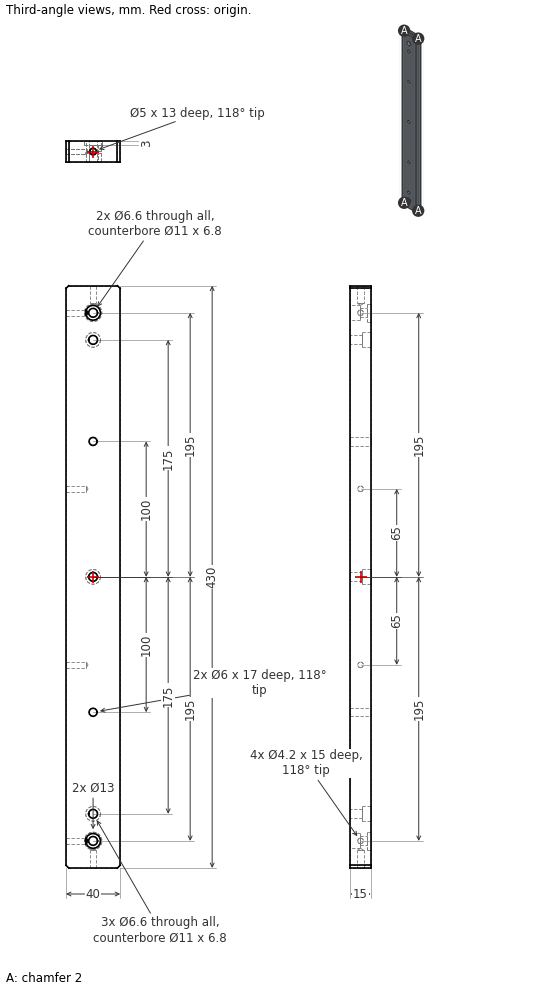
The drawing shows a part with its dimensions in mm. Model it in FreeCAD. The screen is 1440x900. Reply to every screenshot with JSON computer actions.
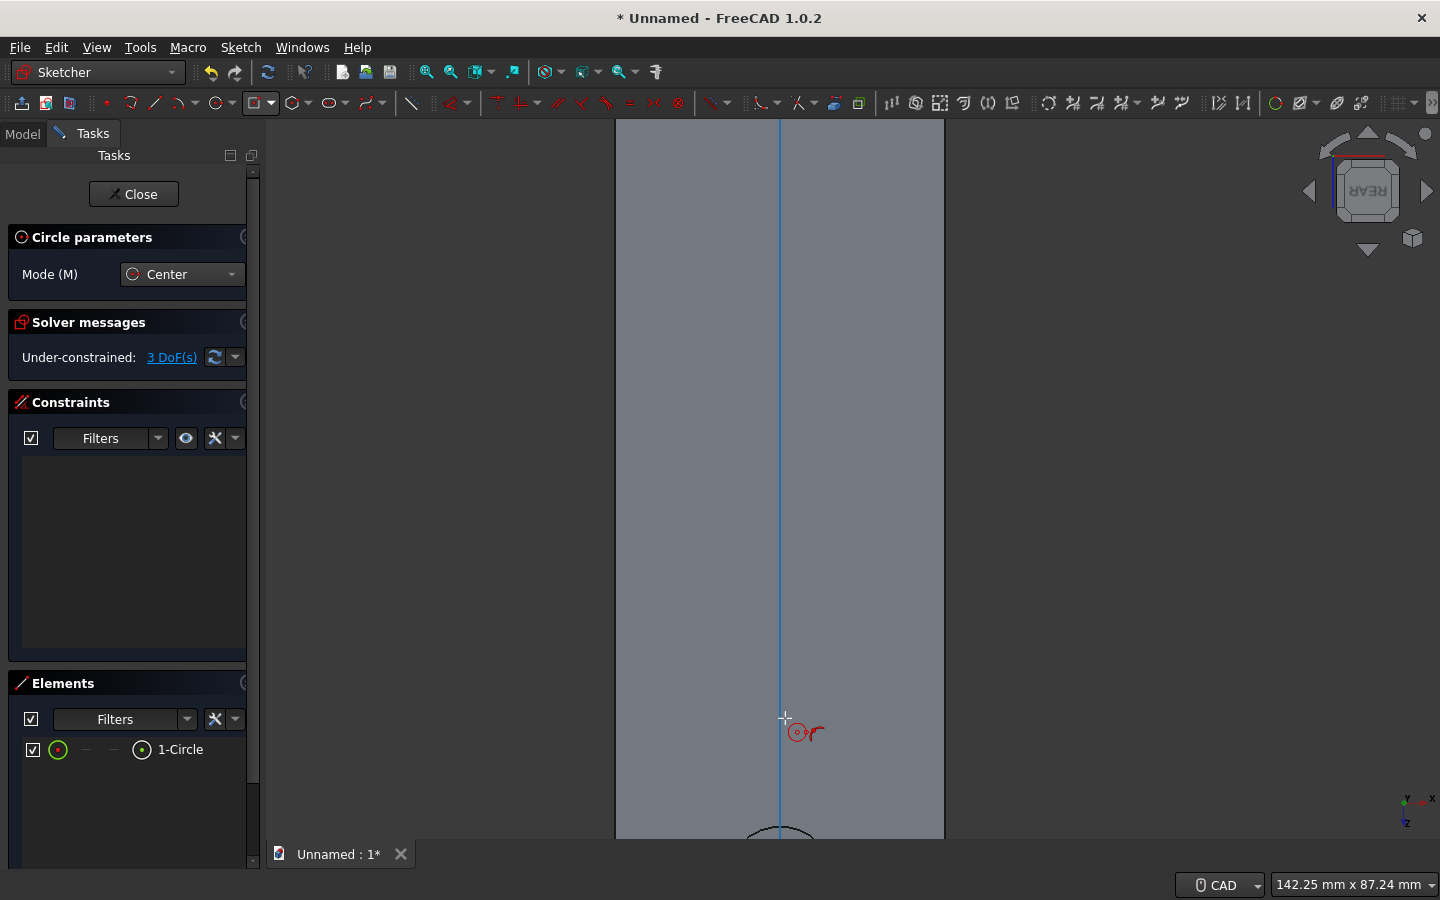
{"action": "scroll", "coordinate": [785, 718], "scroll_direction": "down", "scroll_amount": 9}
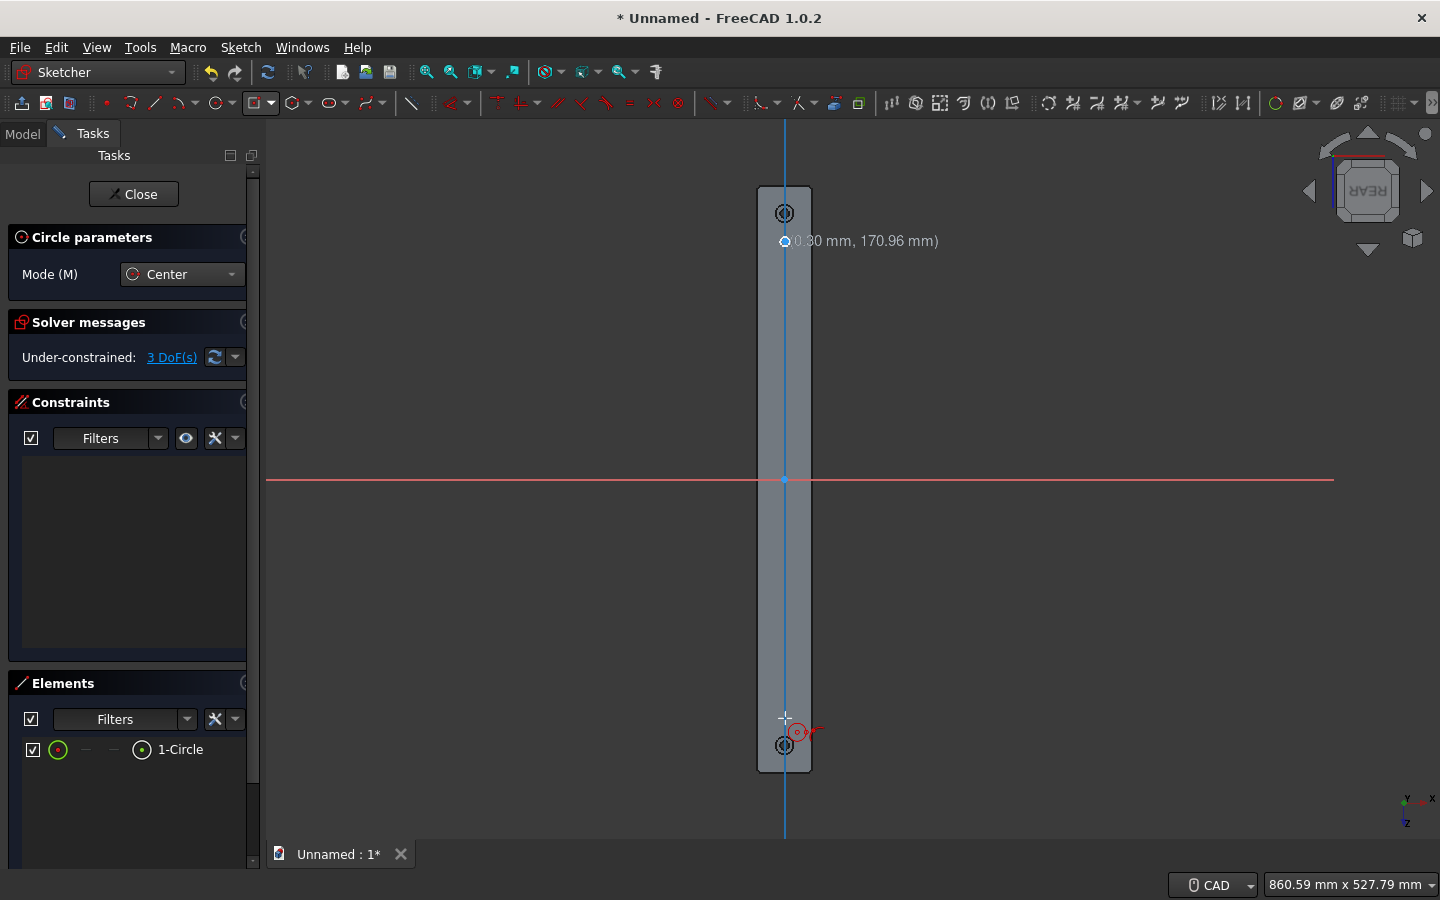
{"action": "left_click", "coordinate": [785, 718]}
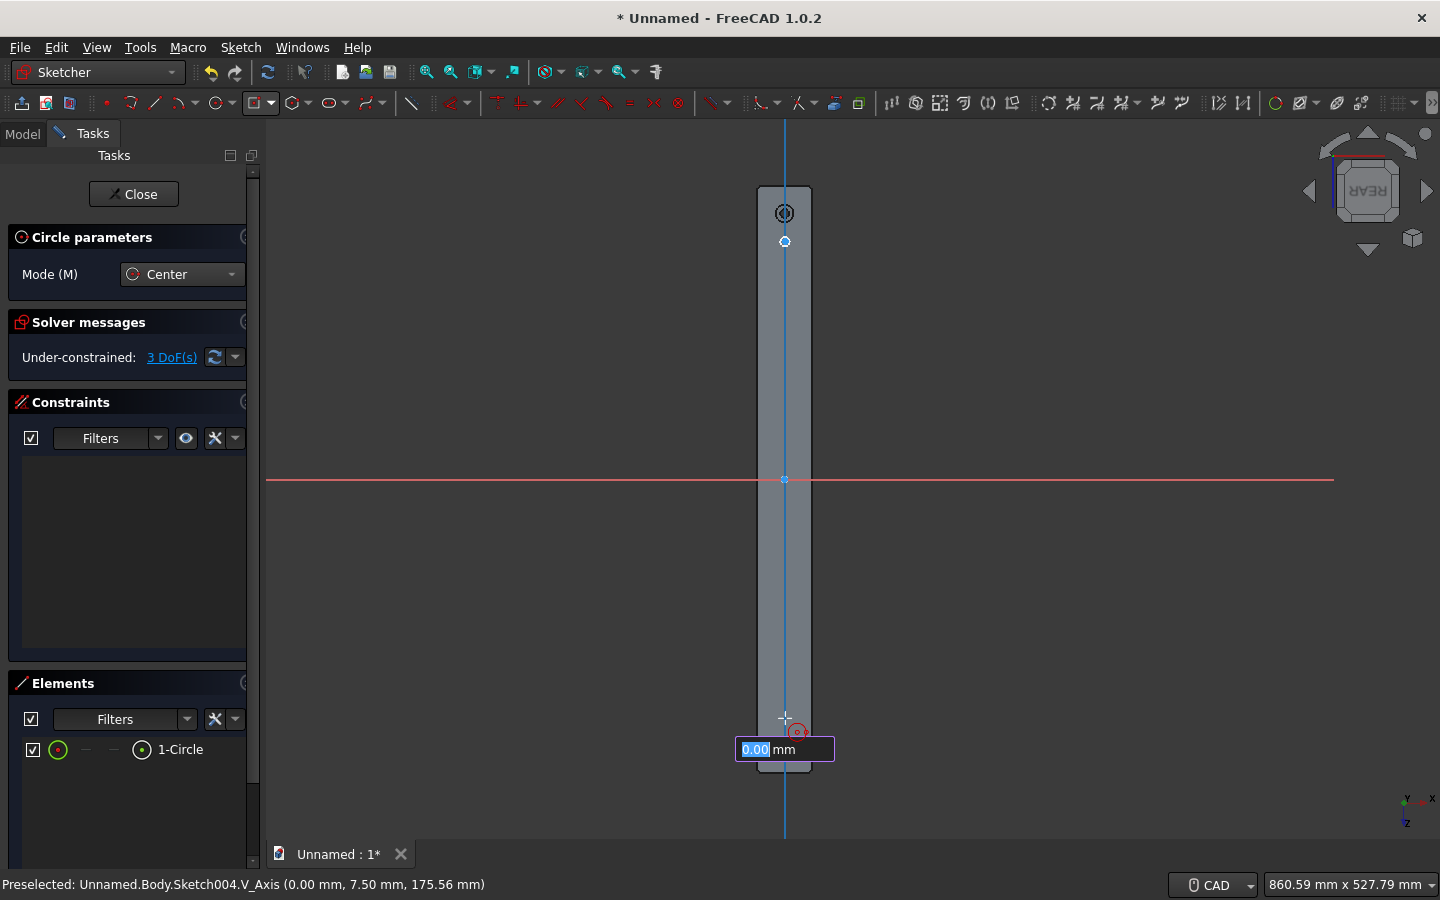
{"action": "scroll", "coordinate": [789, 717], "scroll_direction": "up", "scroll_amount": 7}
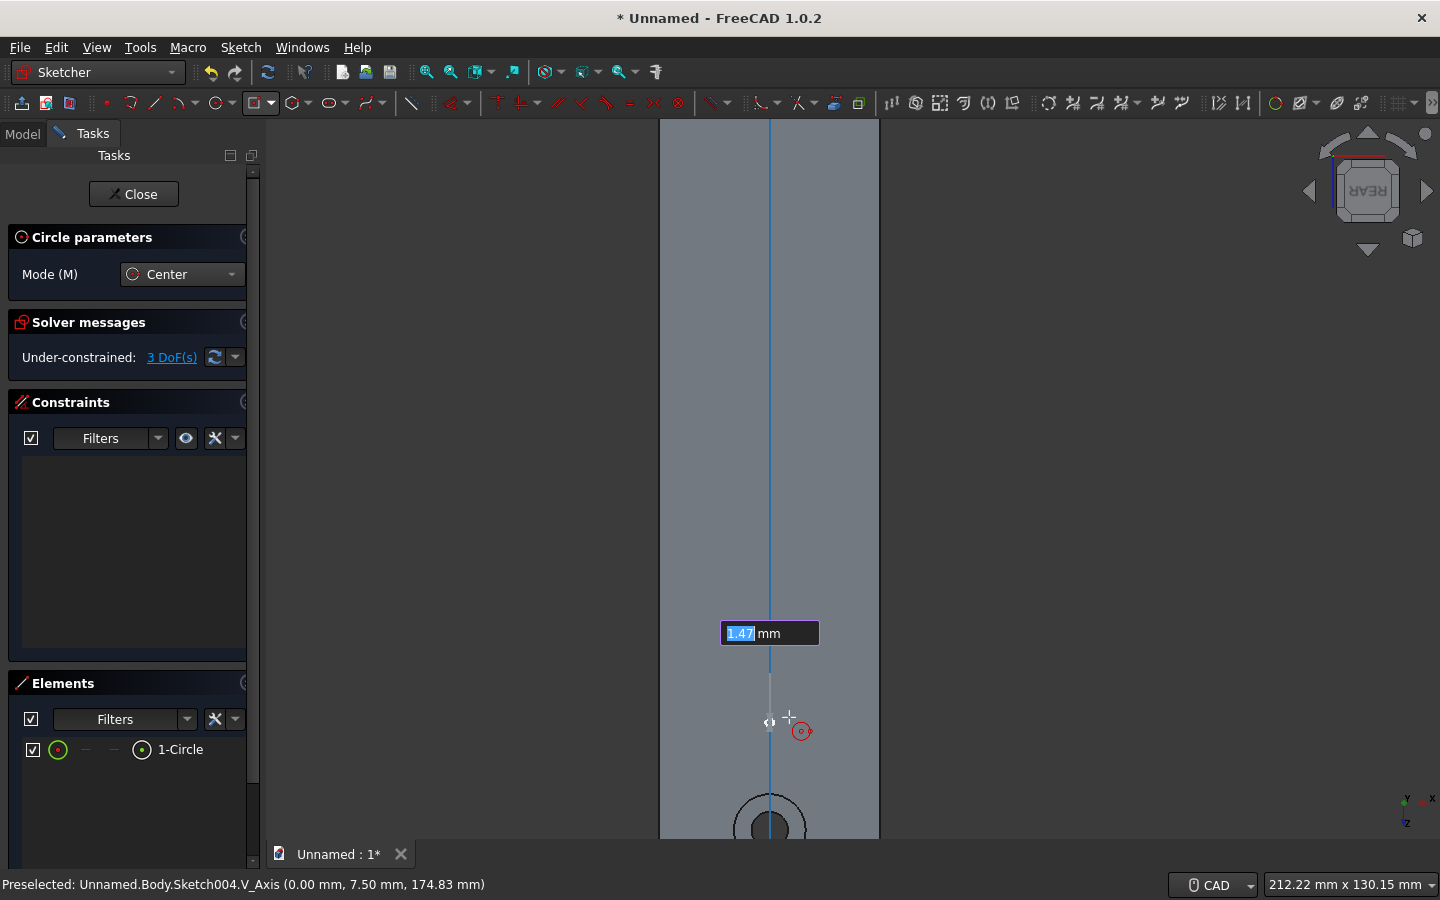
{"action": "left_click", "coordinate": [787, 713]}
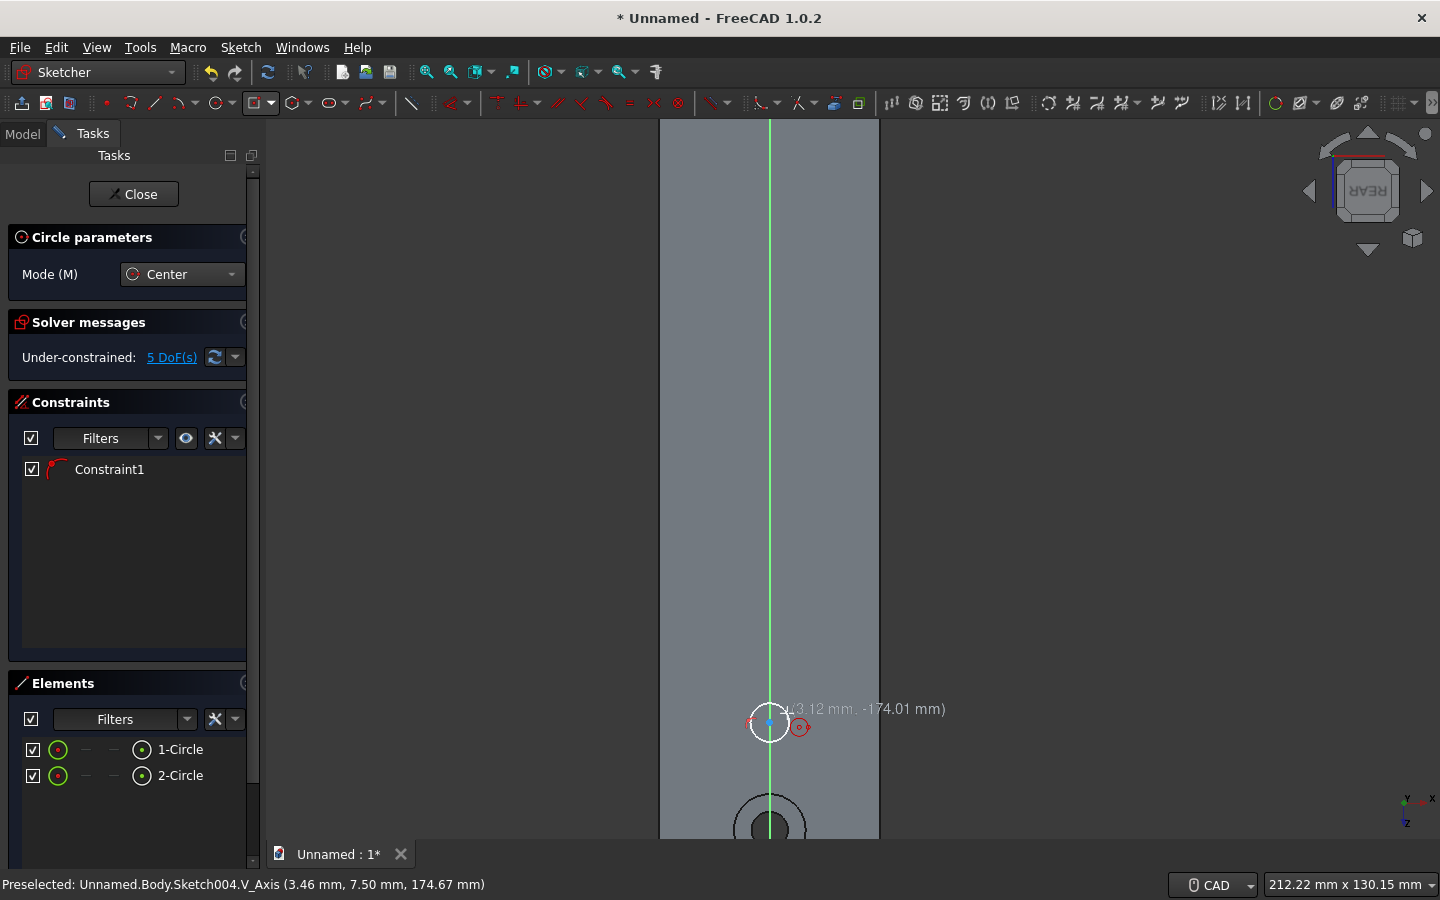
{"action": "scroll", "coordinate": [789, 717], "scroll_direction": "down", "scroll_amount": 7}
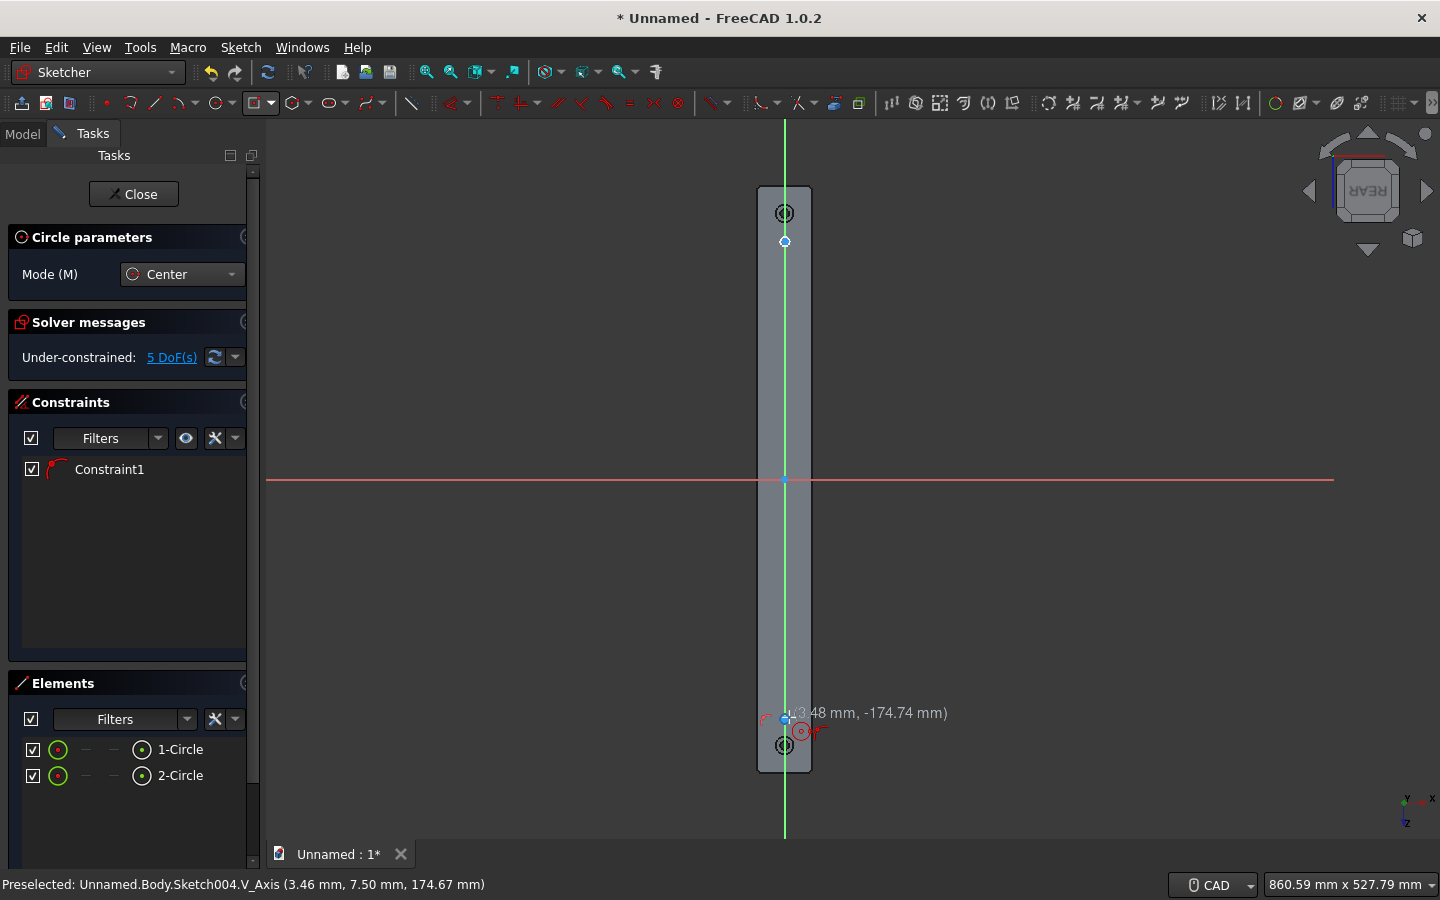
{"action": "scroll", "coordinate": [785, 480], "scroll_direction": "up", "scroll_amount": 9}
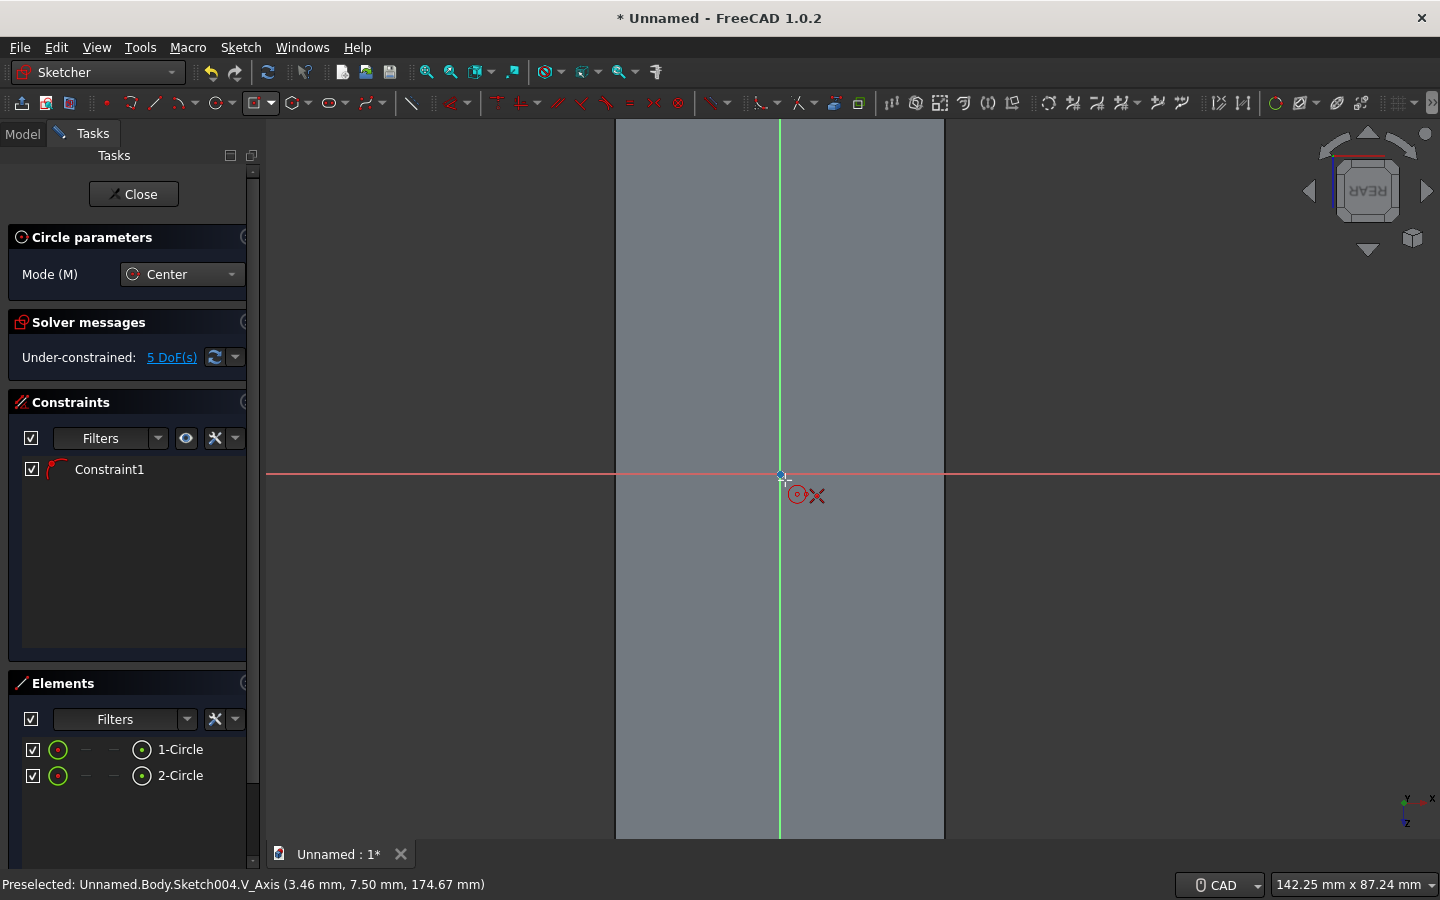
{"action": "scroll", "coordinate": [785, 480], "scroll_direction": "down", "scroll_amount": 9}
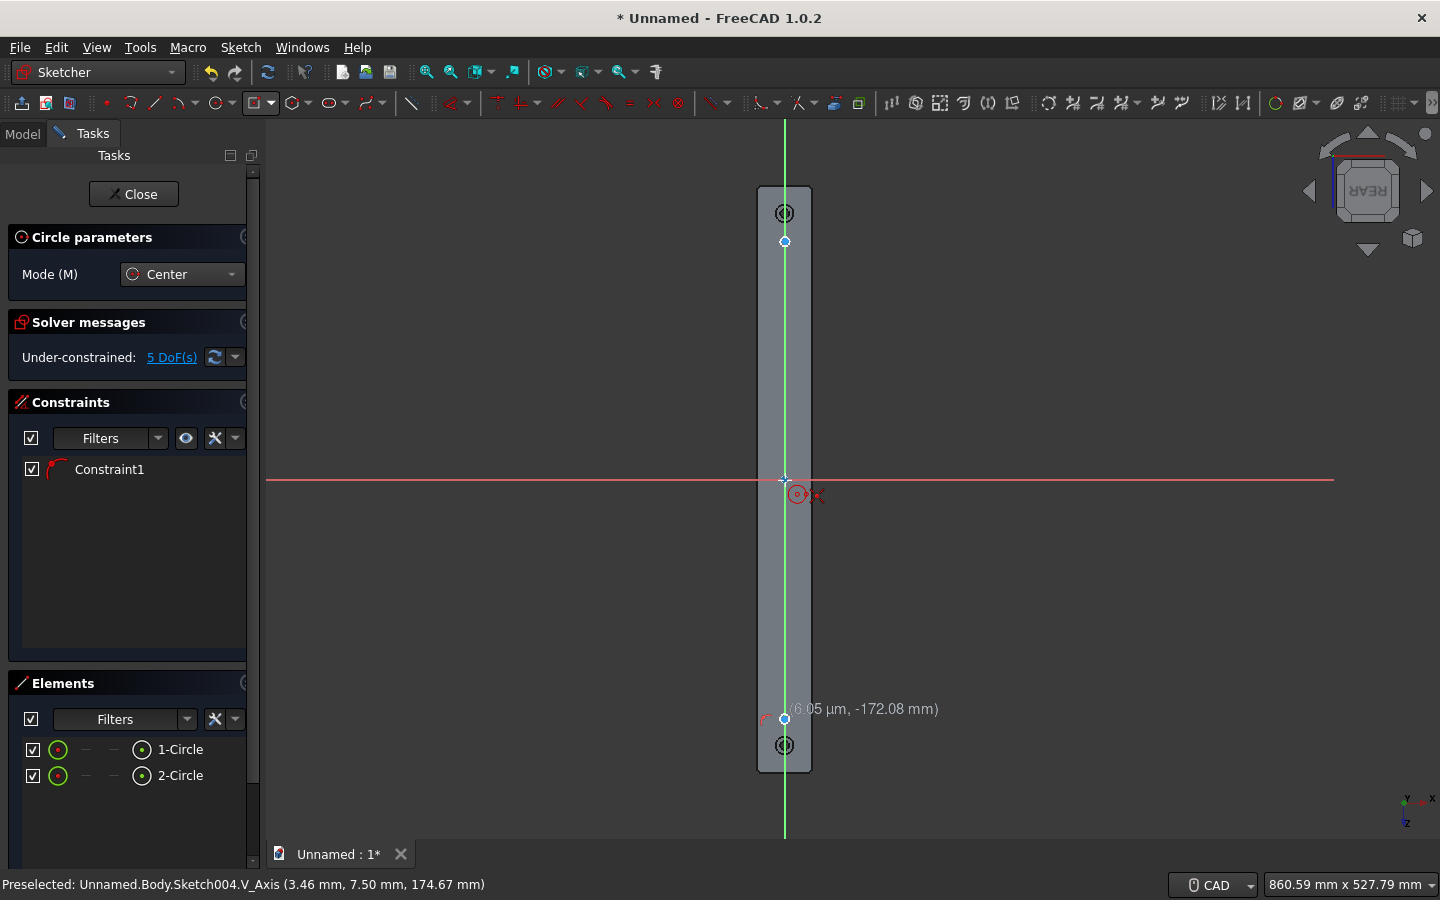
{"action": "left_click", "coordinate": [785, 480]}